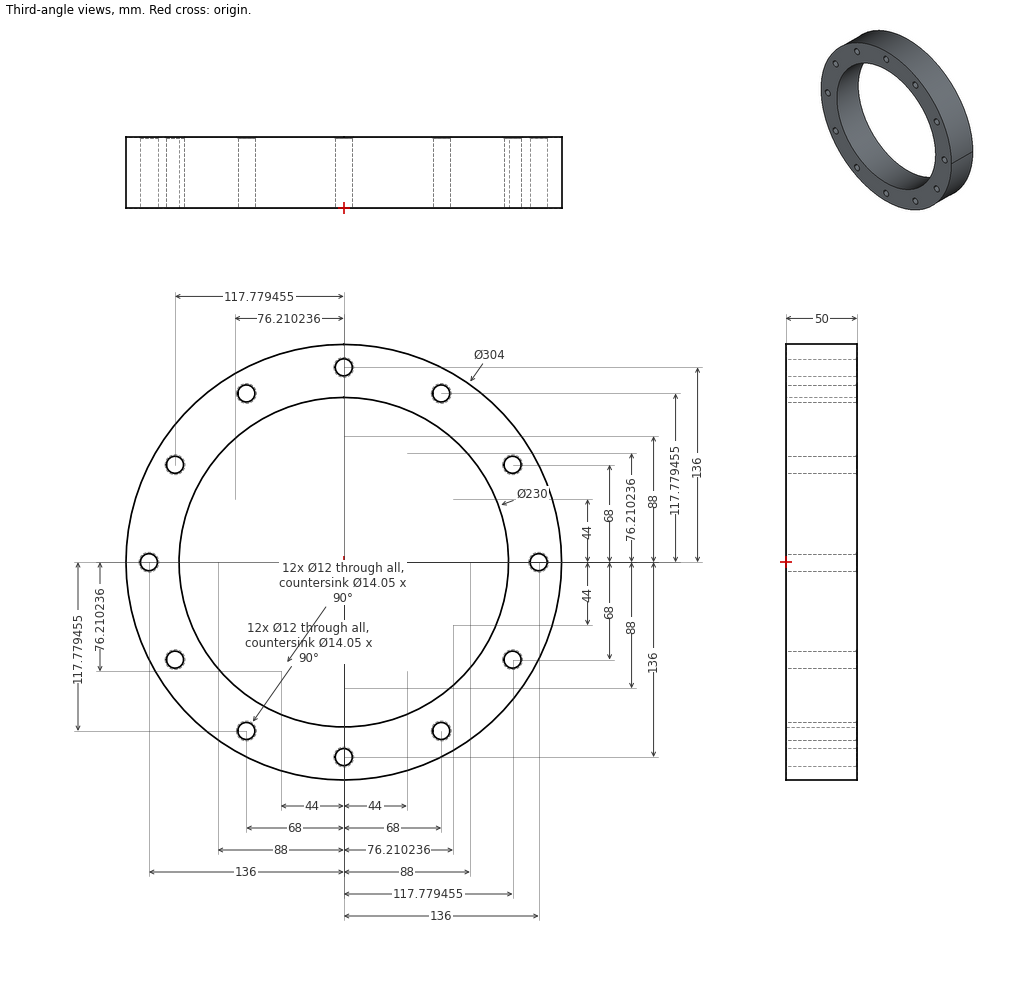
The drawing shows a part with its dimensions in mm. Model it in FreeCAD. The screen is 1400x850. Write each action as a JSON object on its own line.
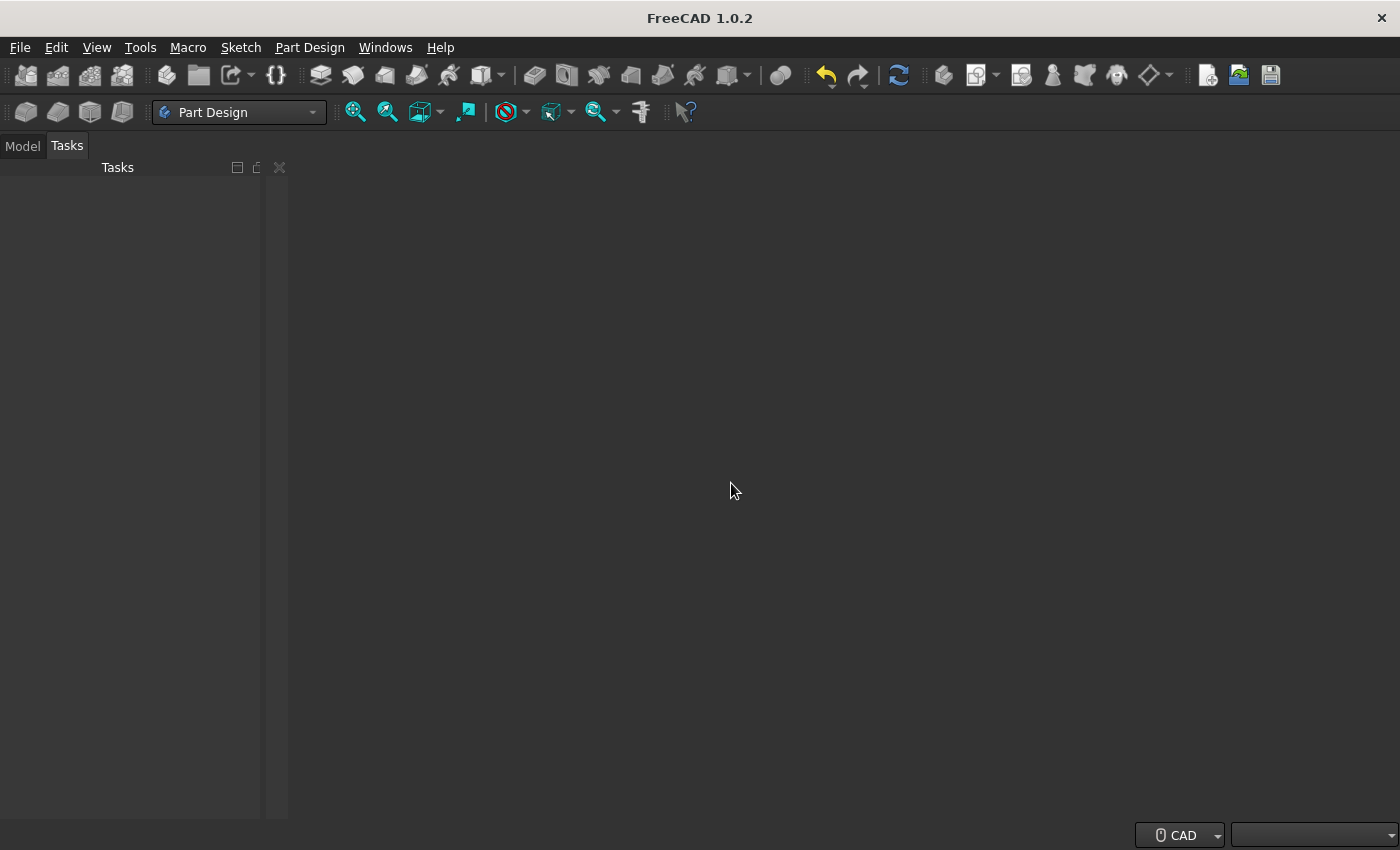
{"action": "left_click", "coordinate": [1208, 76]}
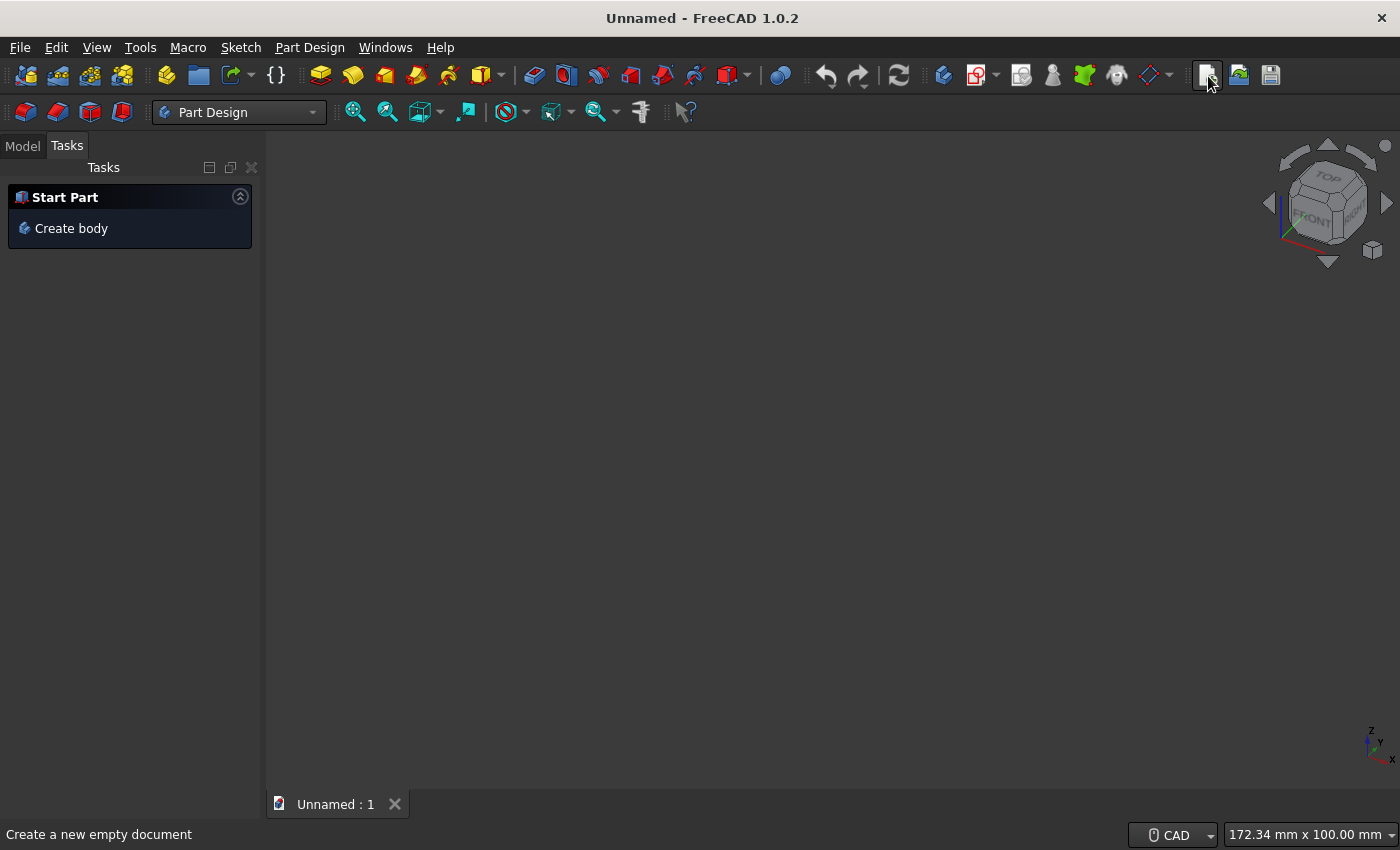
{"action": "left_click", "coordinate": [976, 76]}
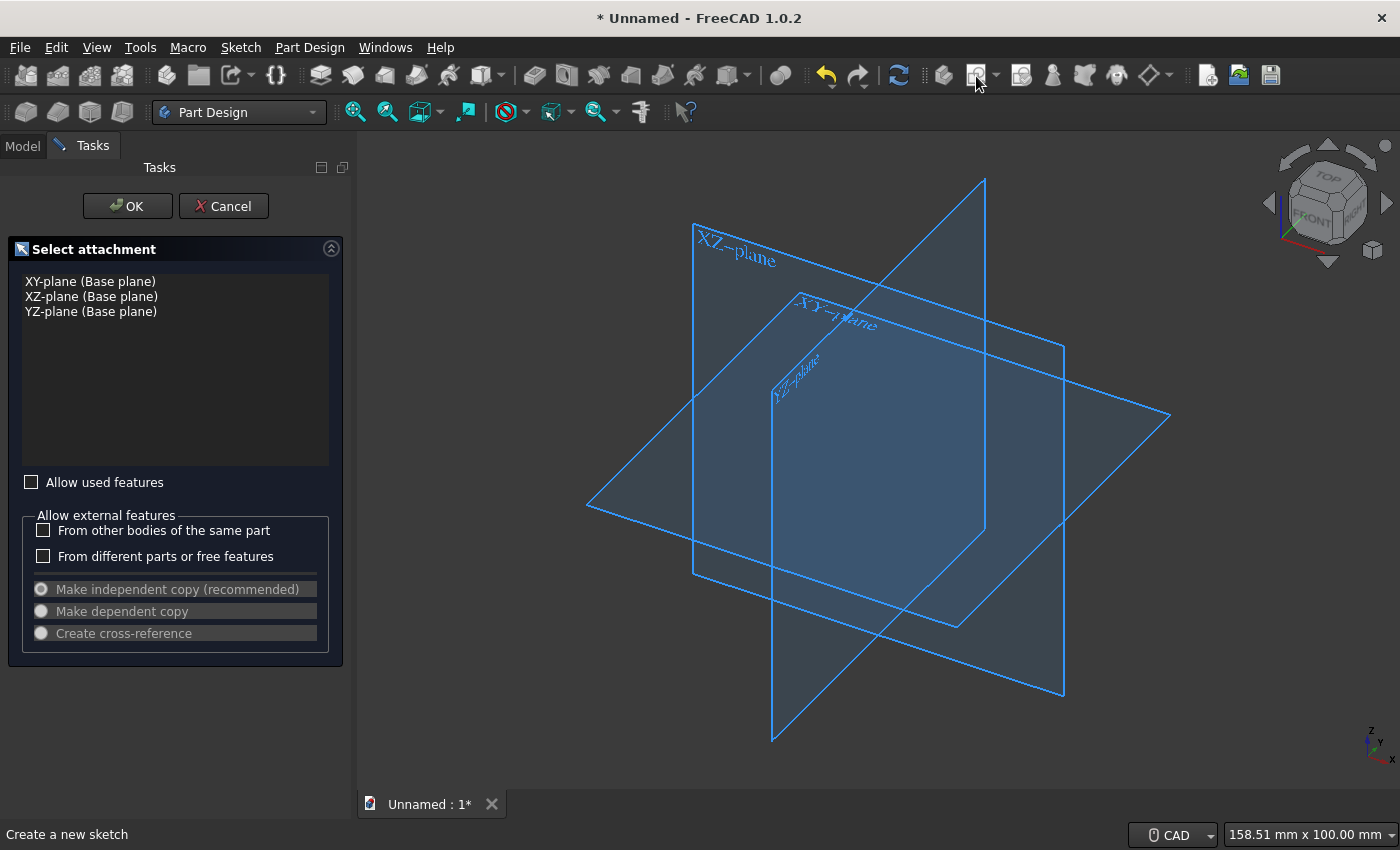
{"action": "left_click", "coordinate": [82, 296]}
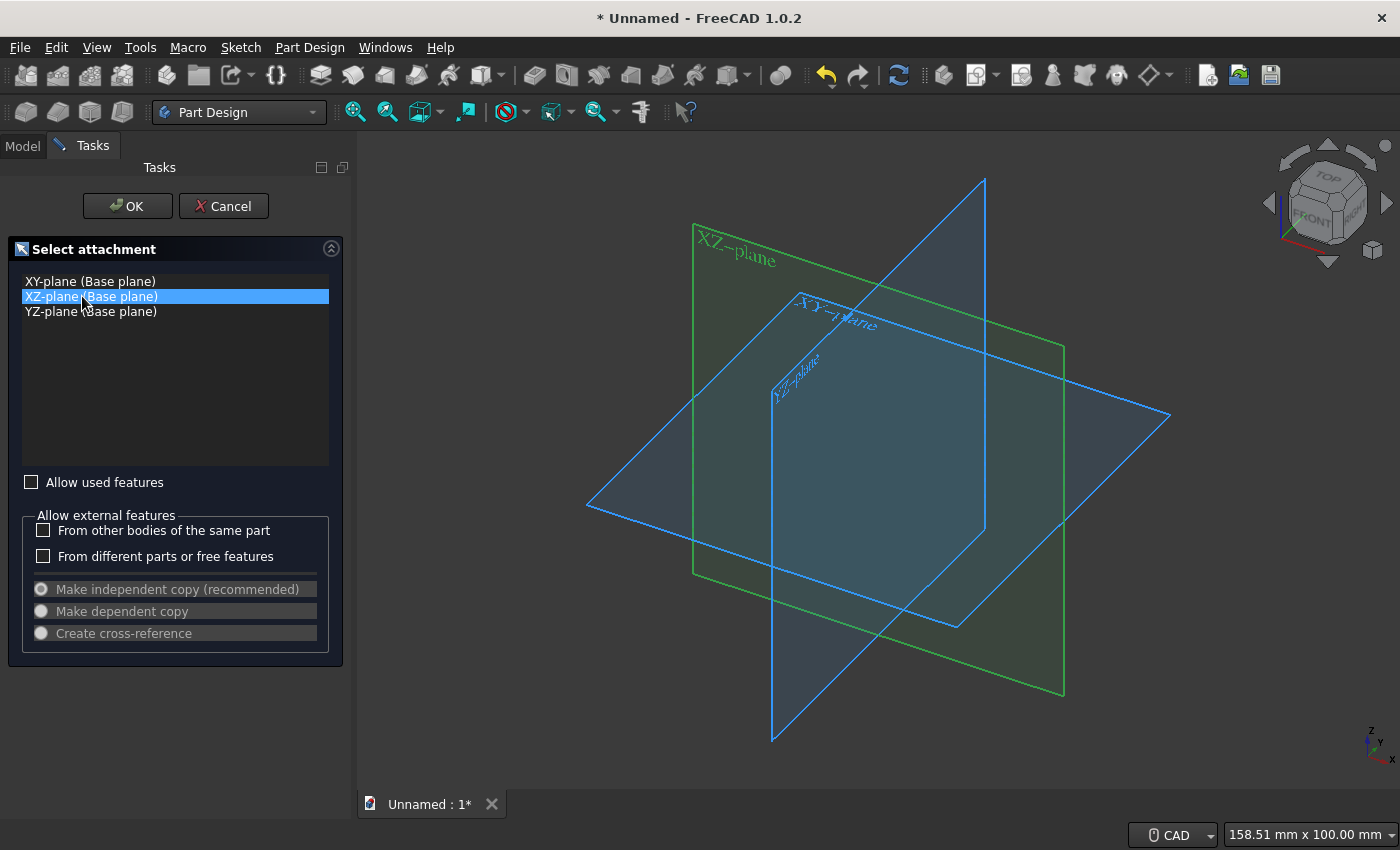
{"action": "left_click", "coordinate": [128, 206]}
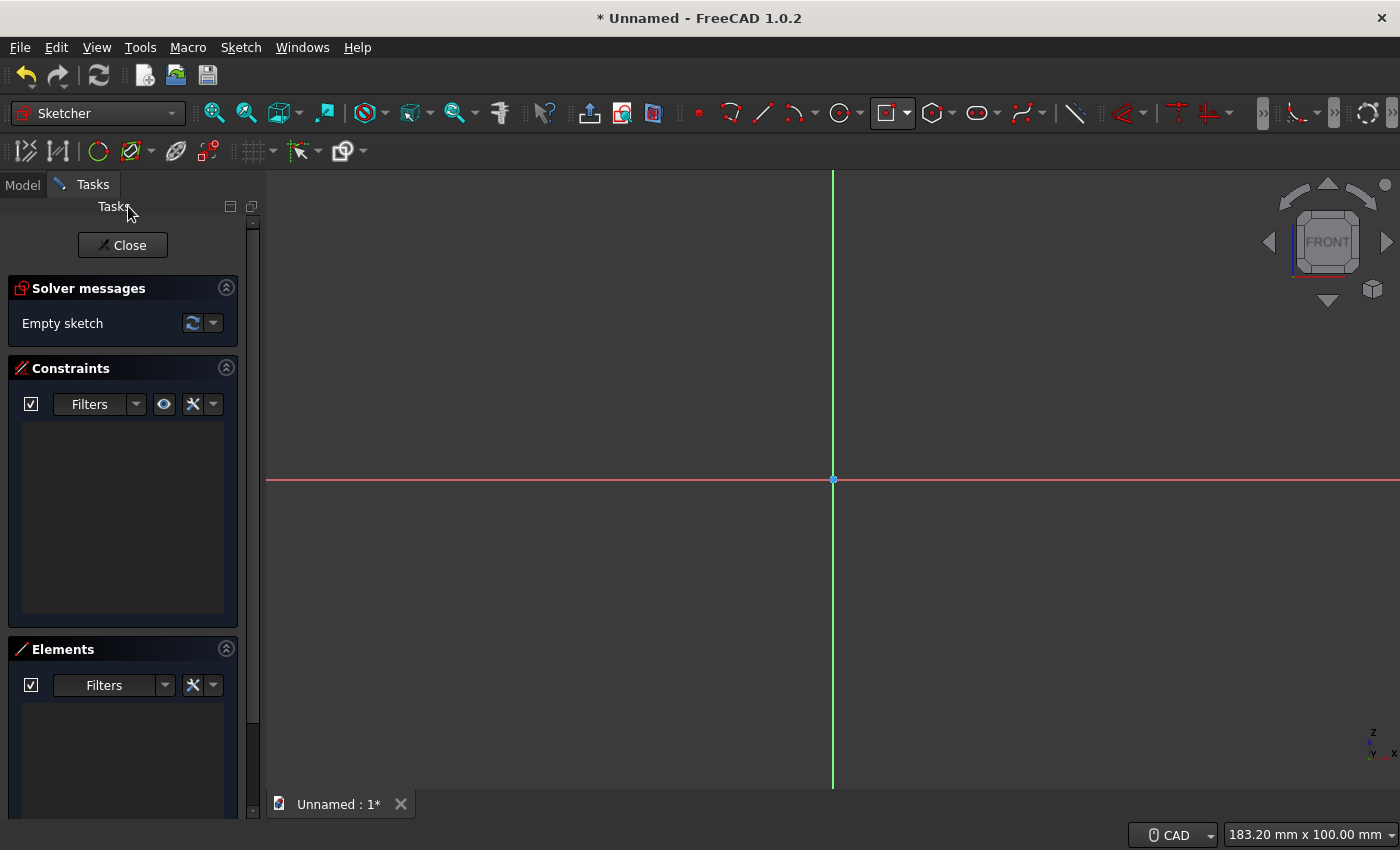
{"action": "scroll", "coordinate": [747, 480], "scroll_direction": "down", "scroll_amount": 8}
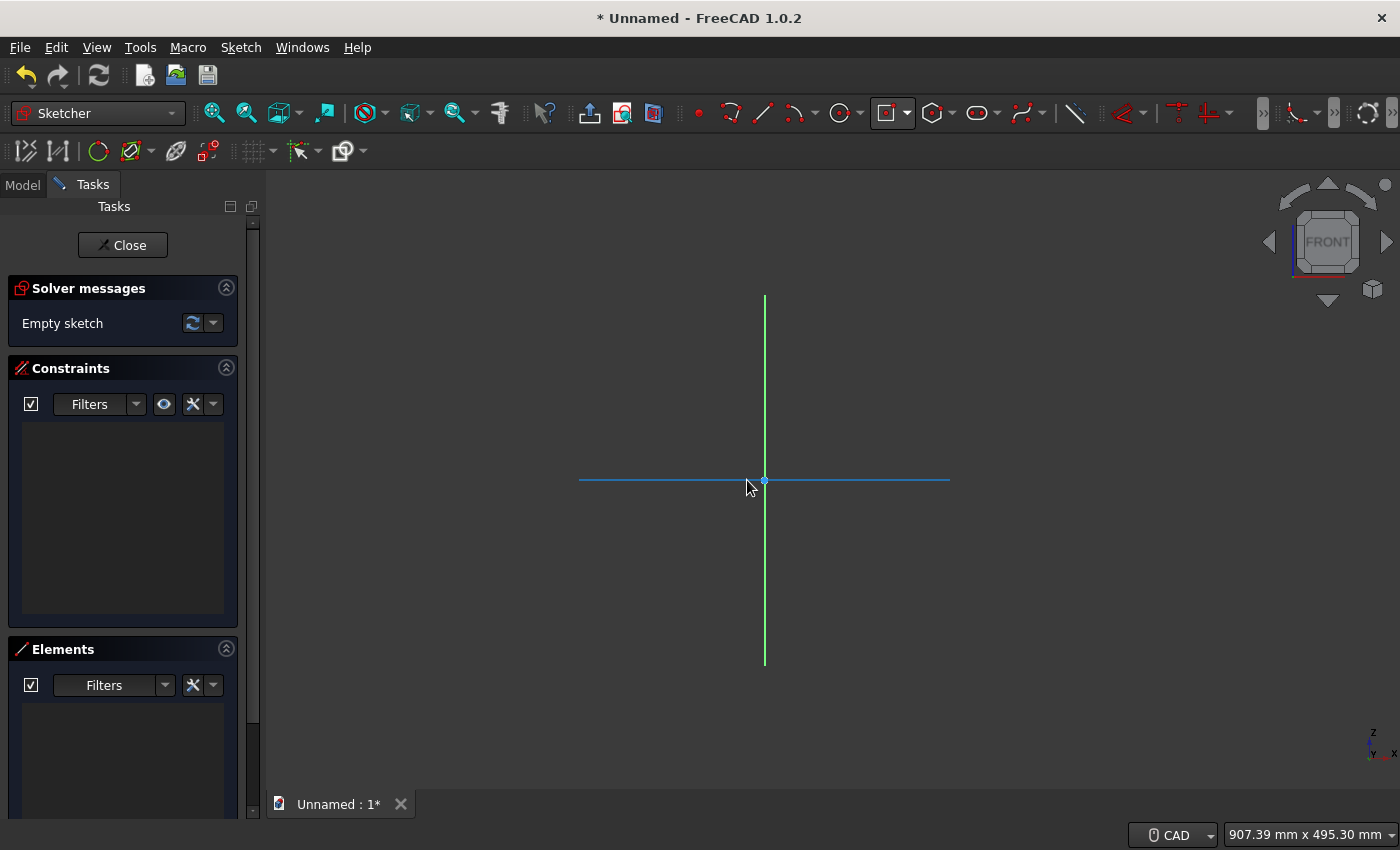
{"action": "left_click", "coordinate": [840, 114]}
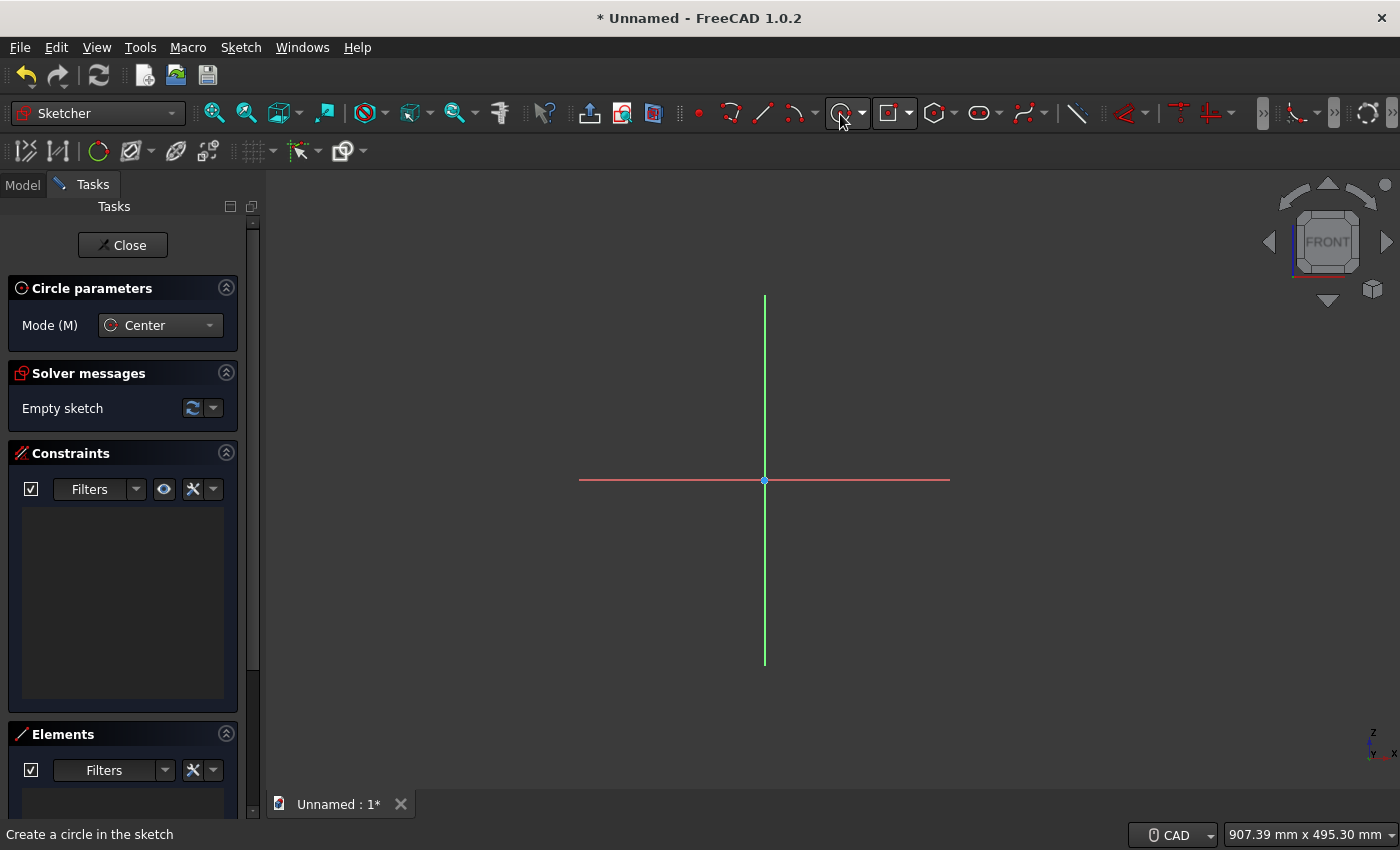
{"action": "left_click", "coordinate": [765, 480]}
{"action": "left_click", "coordinate": [899, 346]}
{"action": "key", "text": "Escape"}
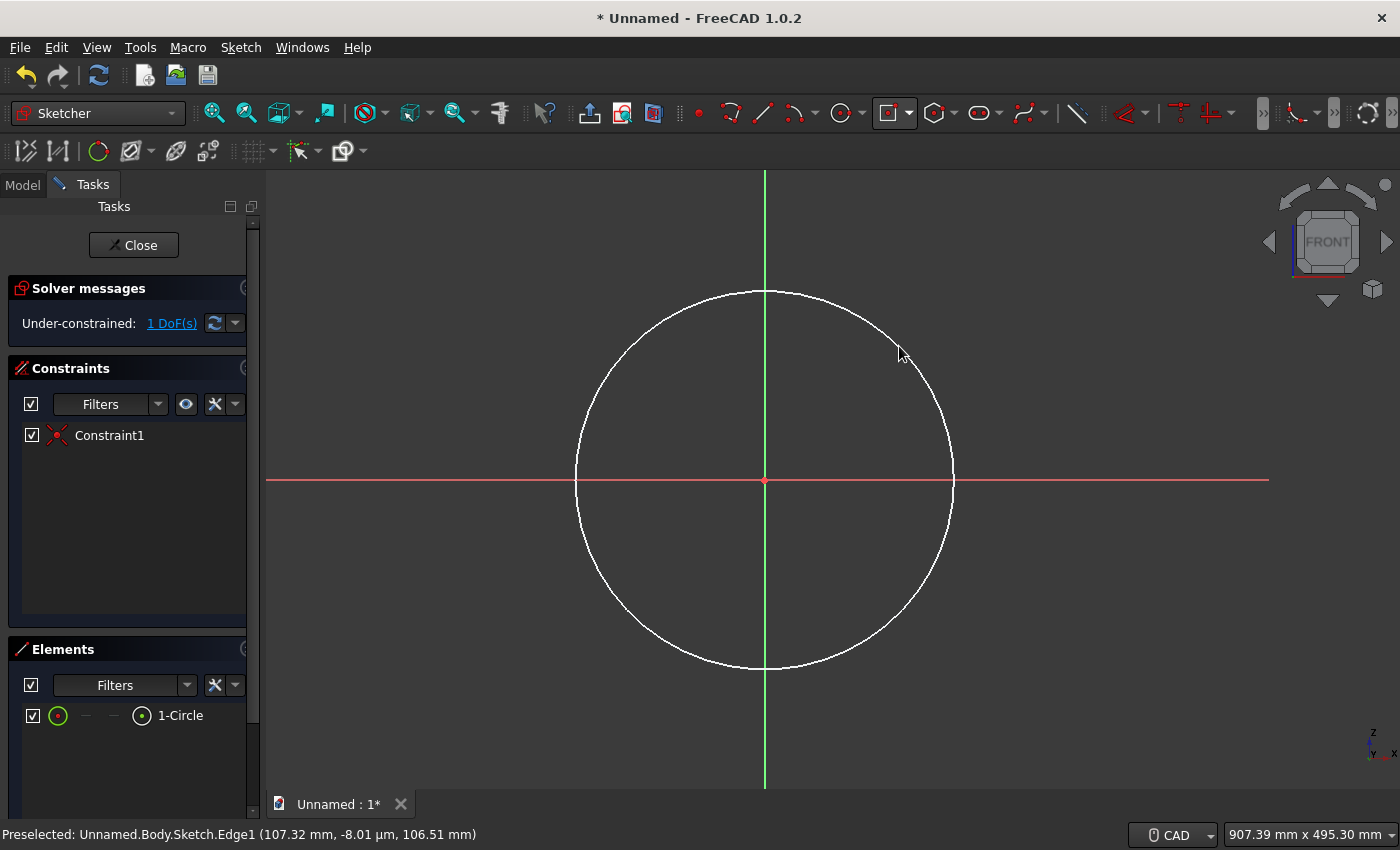
{"action": "left_click", "coordinate": [1124, 114]}